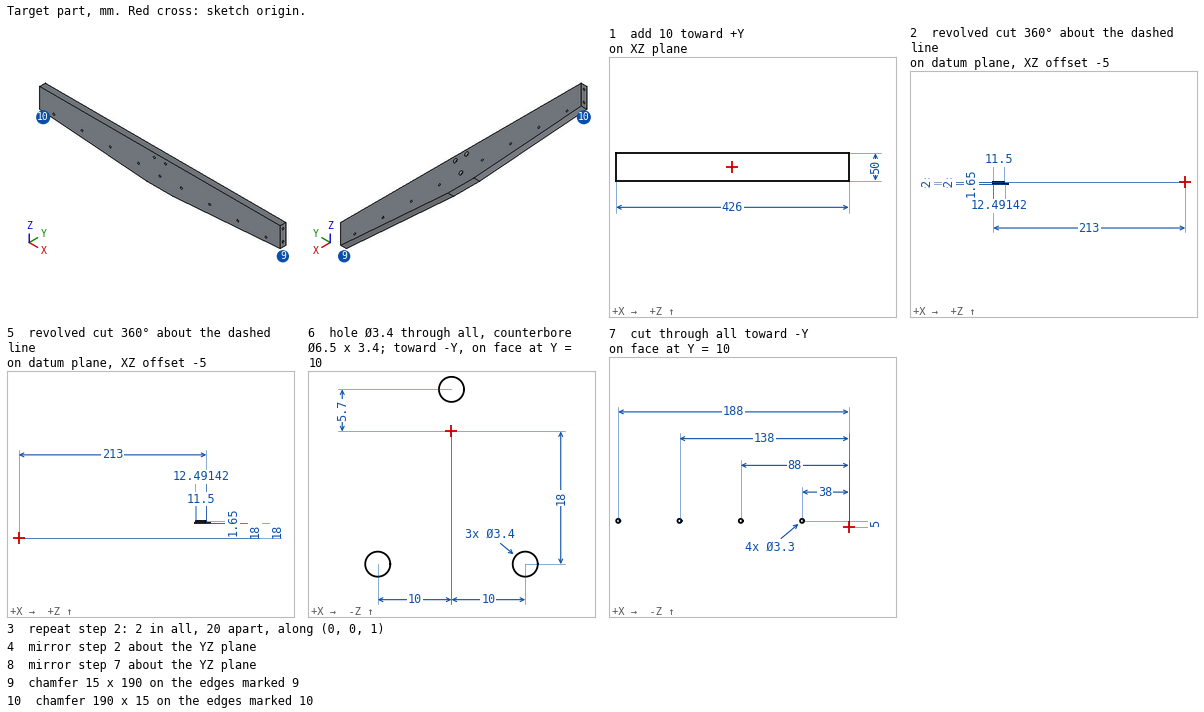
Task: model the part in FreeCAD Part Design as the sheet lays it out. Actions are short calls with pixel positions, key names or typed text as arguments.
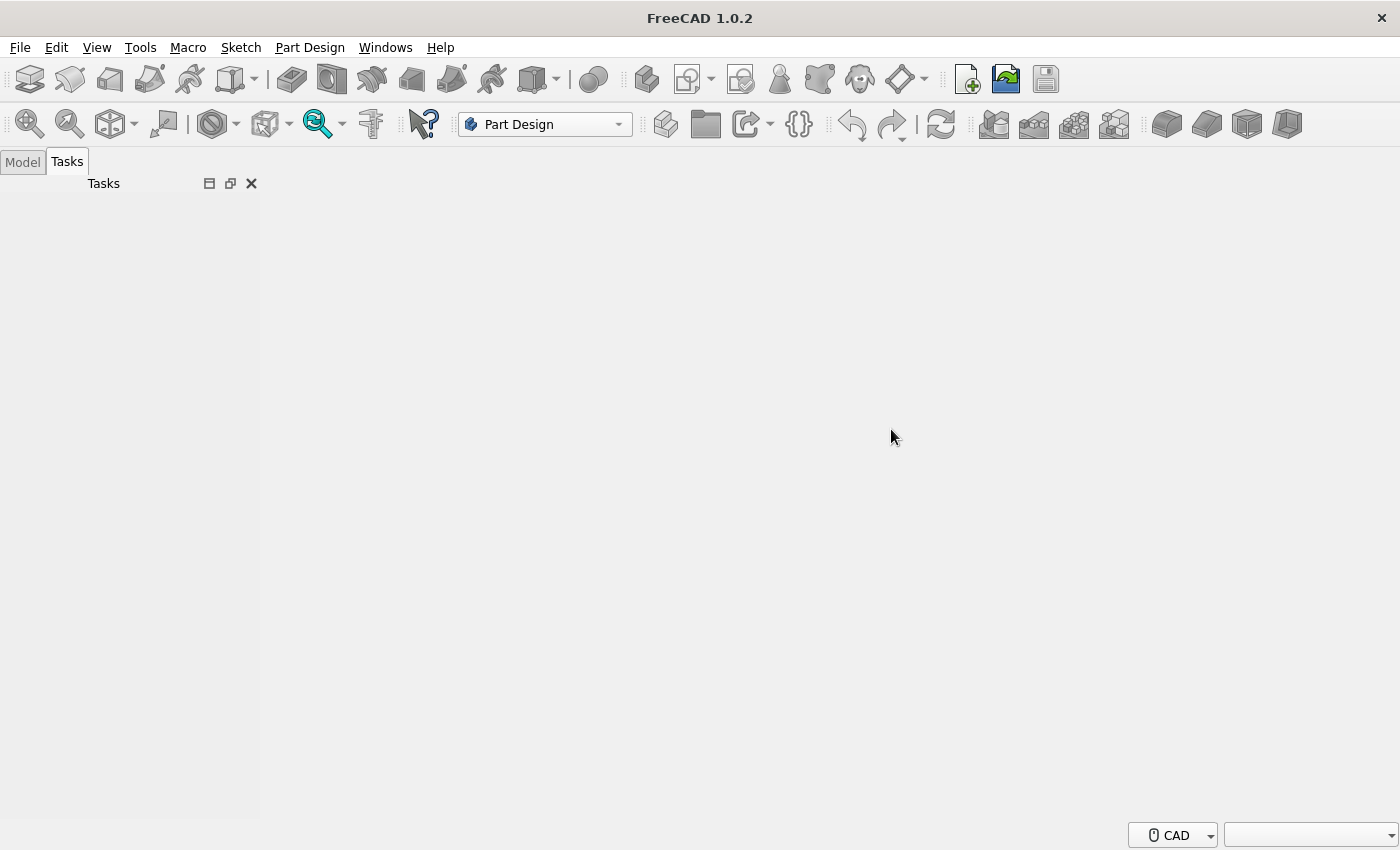
click(966, 80)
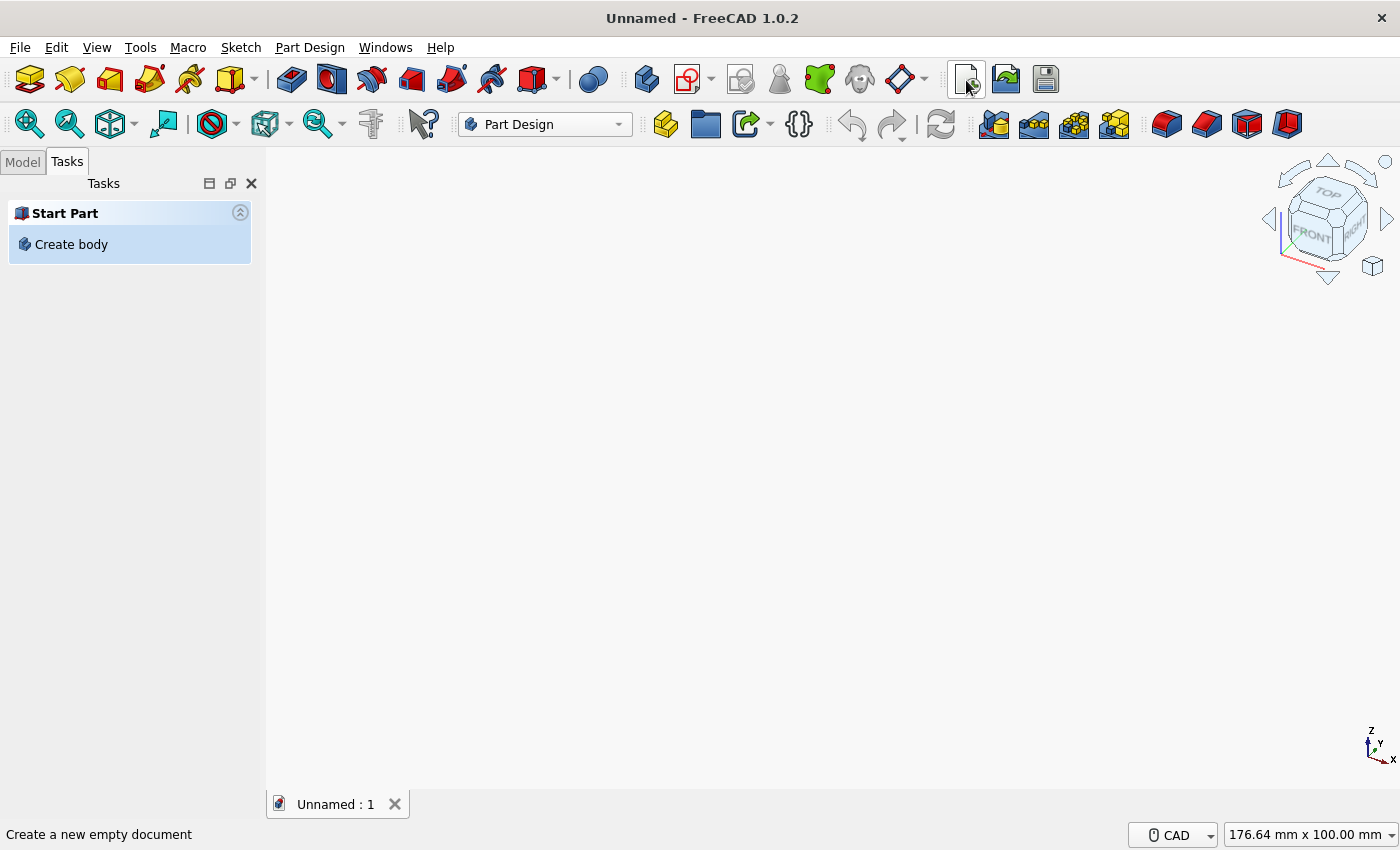
click(688, 80)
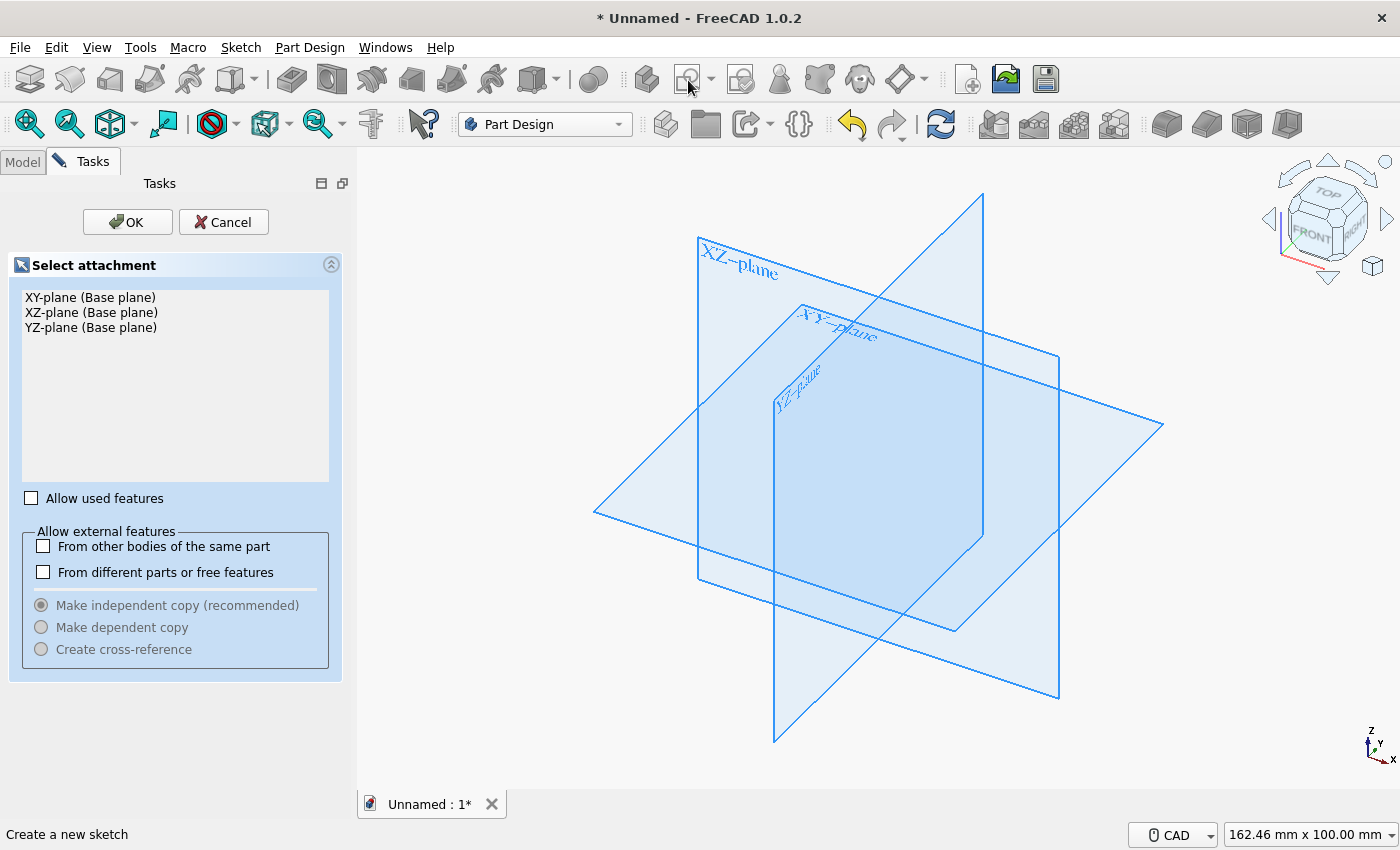
click(82, 312)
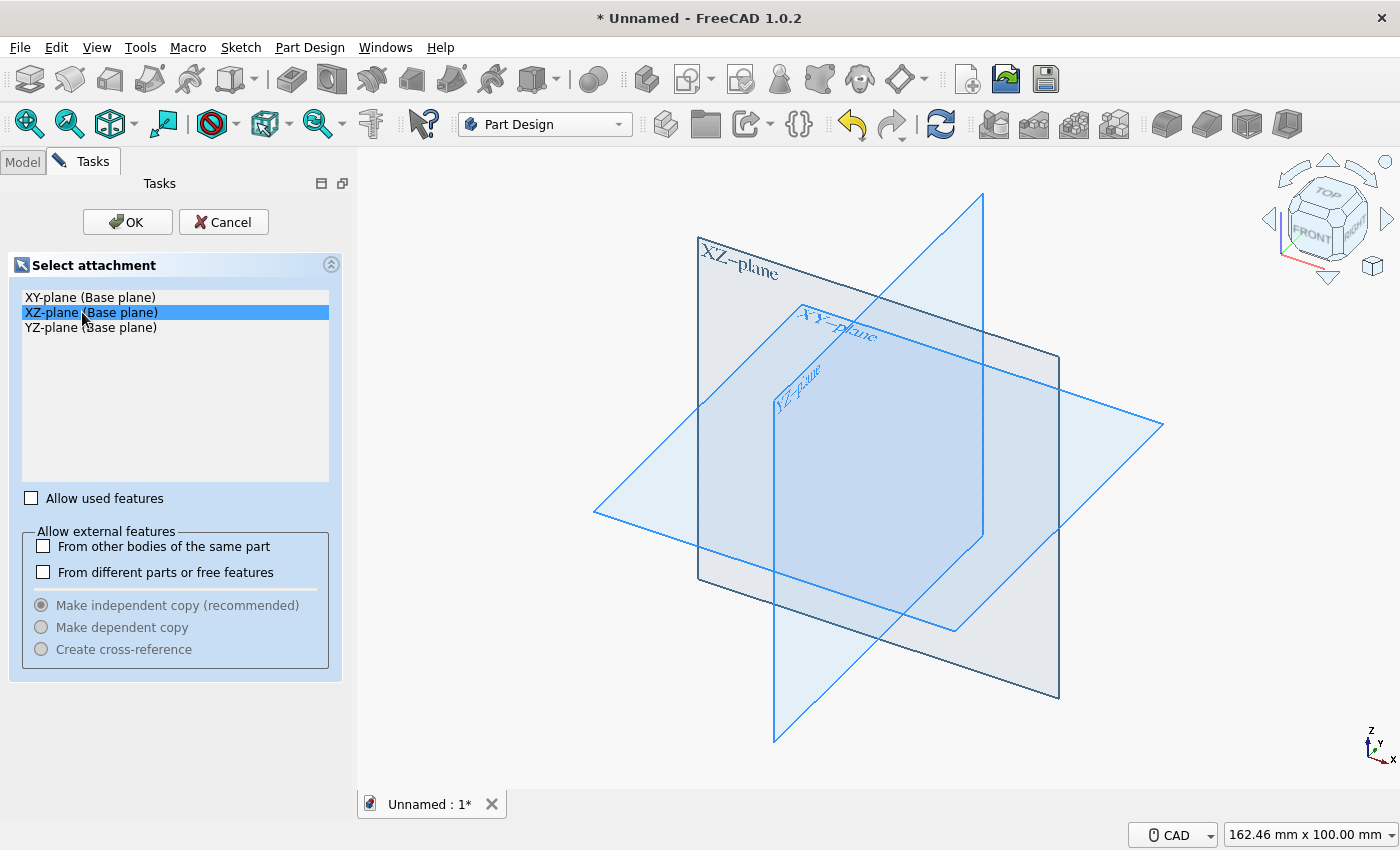
click(128, 222)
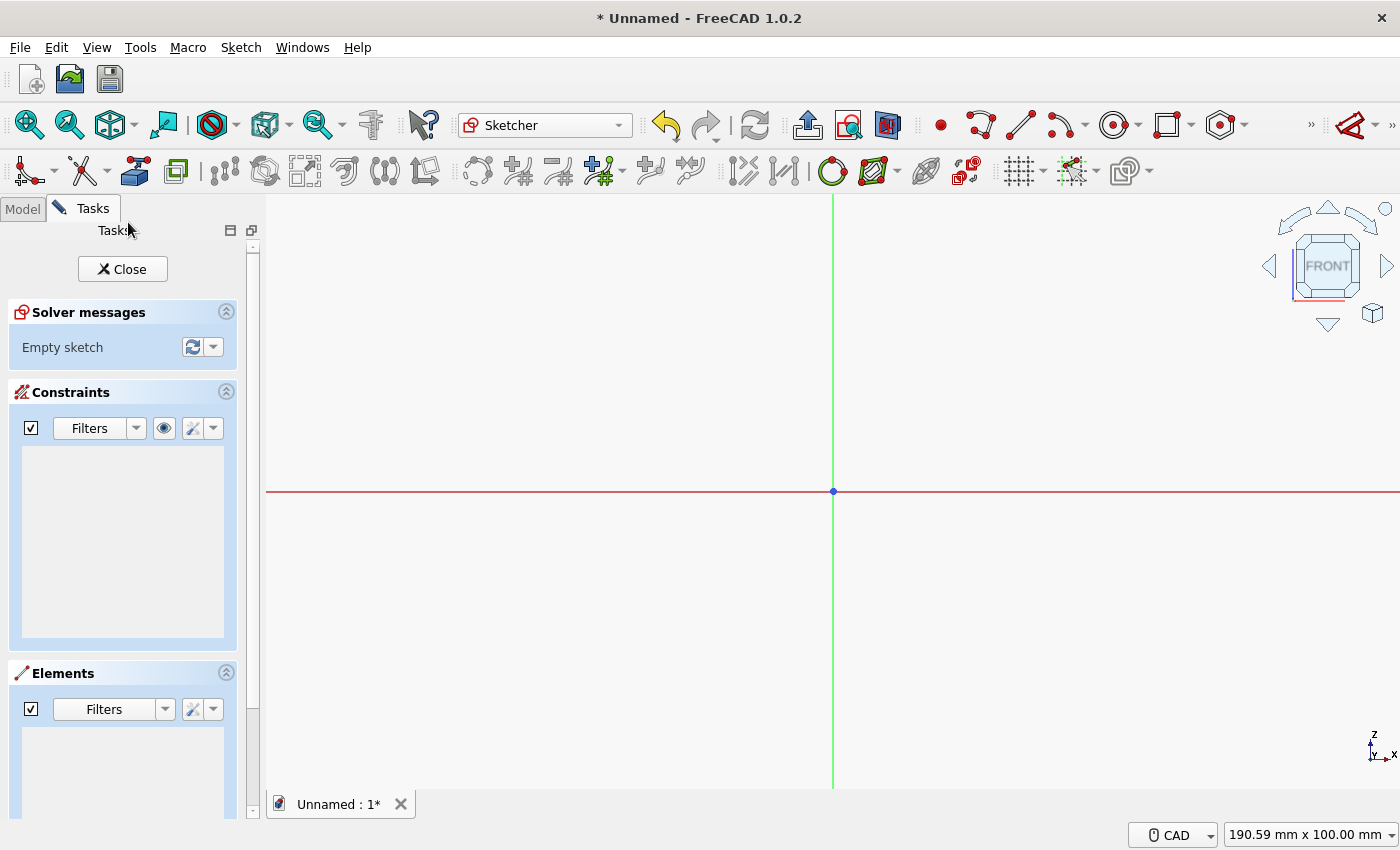
scroll(742, 492, down, 7)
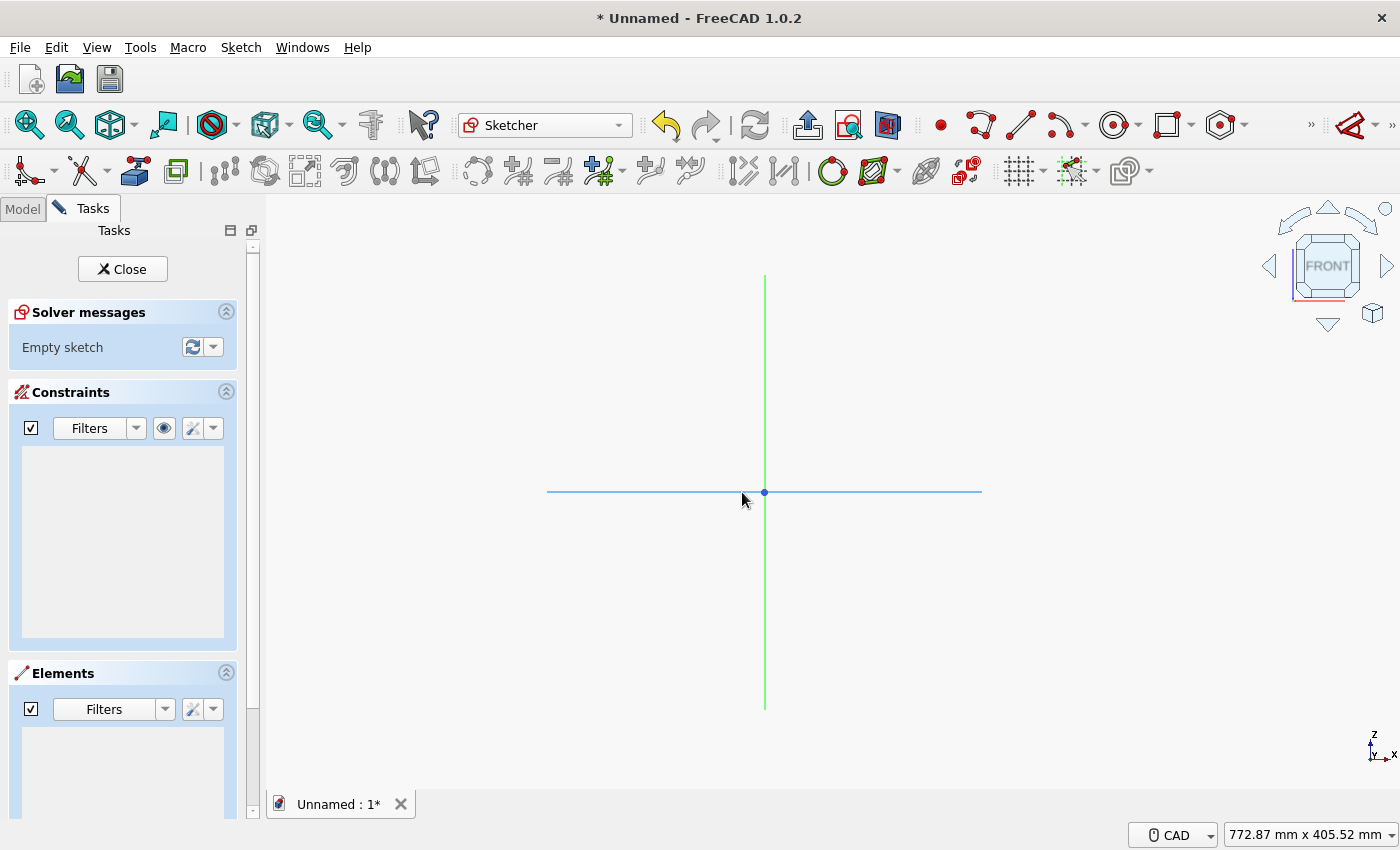
click(1194, 126)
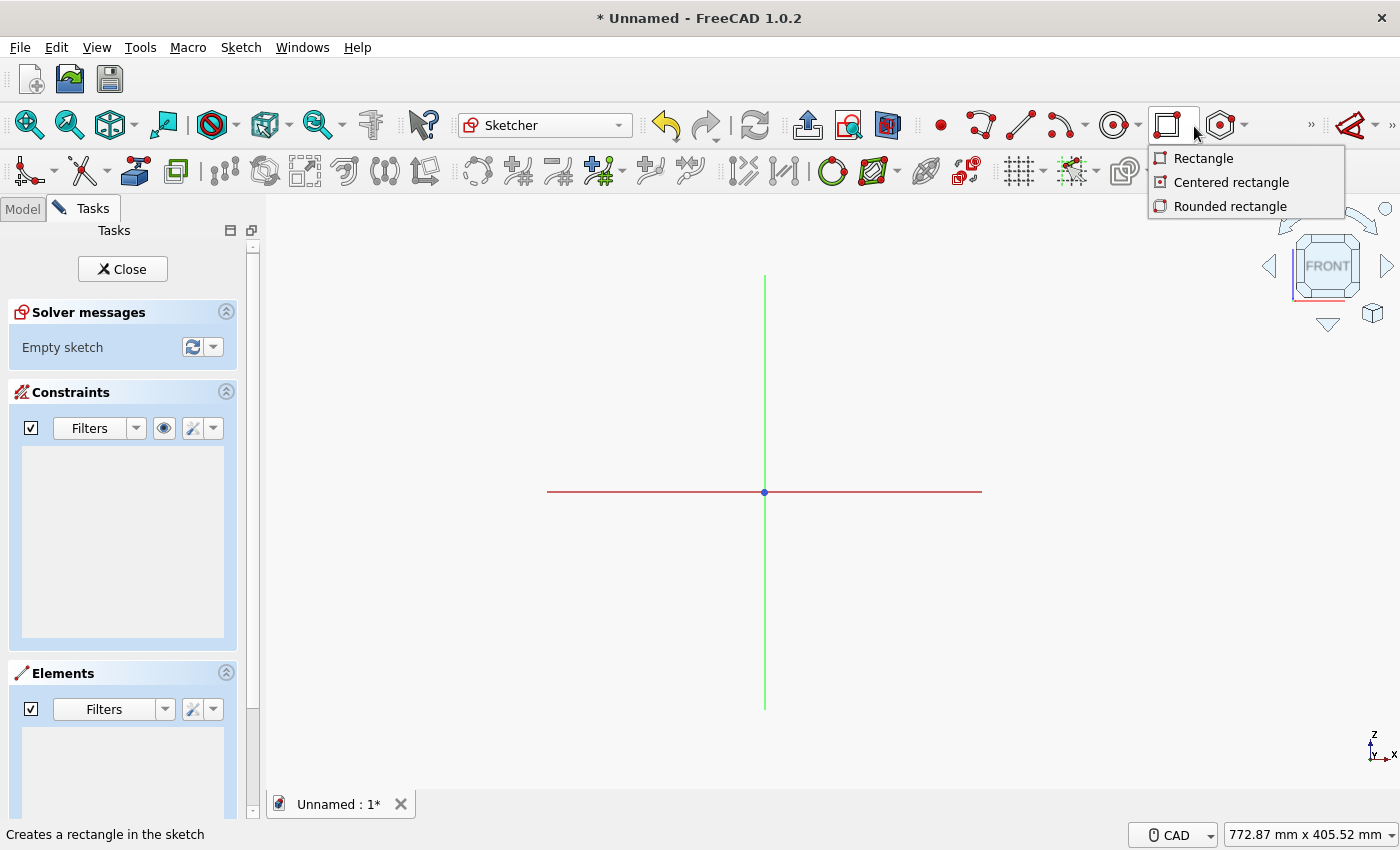
click(1246, 182)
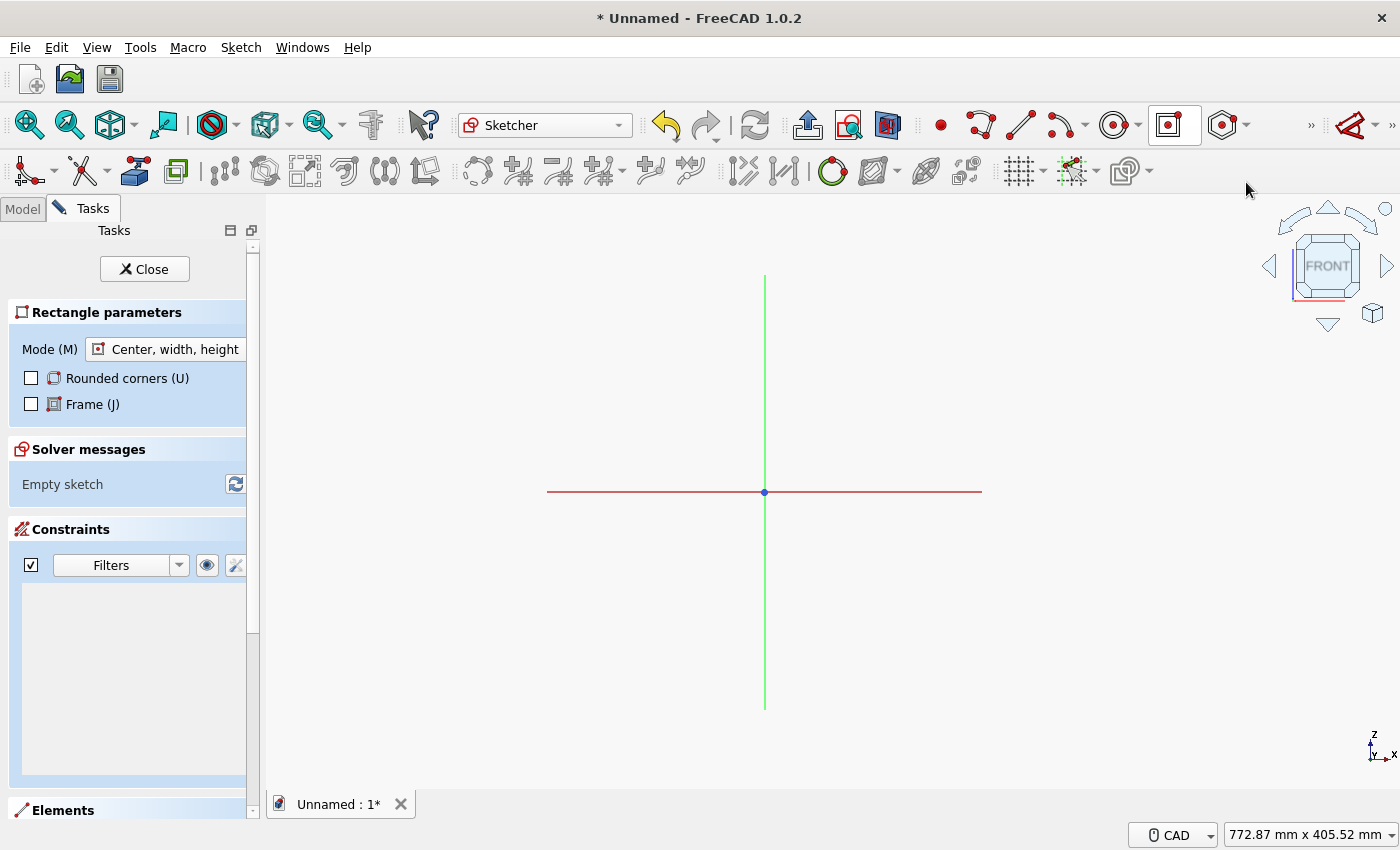
click(765, 492)
move(1077, 456)